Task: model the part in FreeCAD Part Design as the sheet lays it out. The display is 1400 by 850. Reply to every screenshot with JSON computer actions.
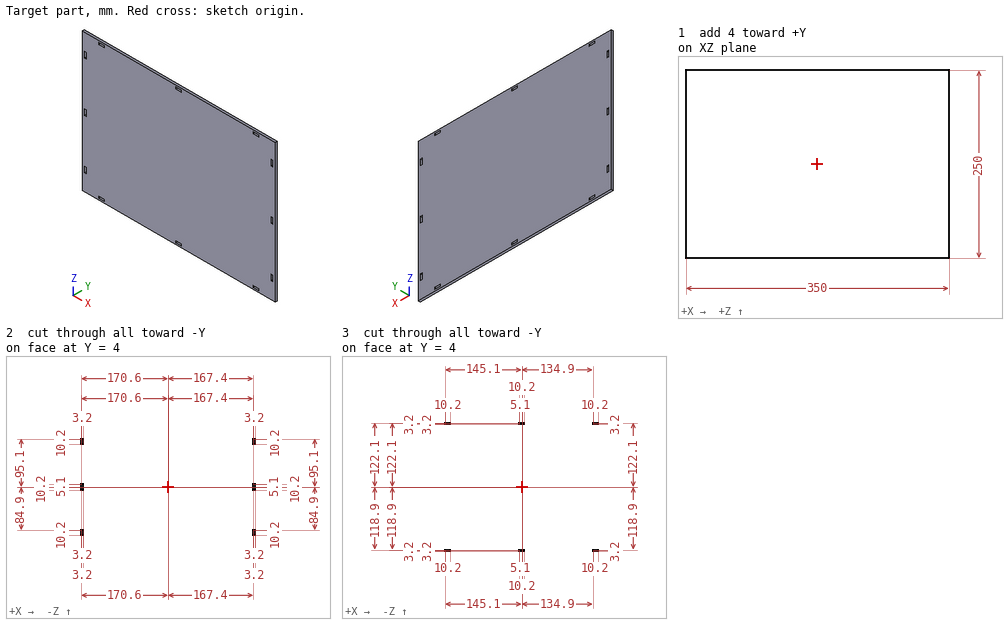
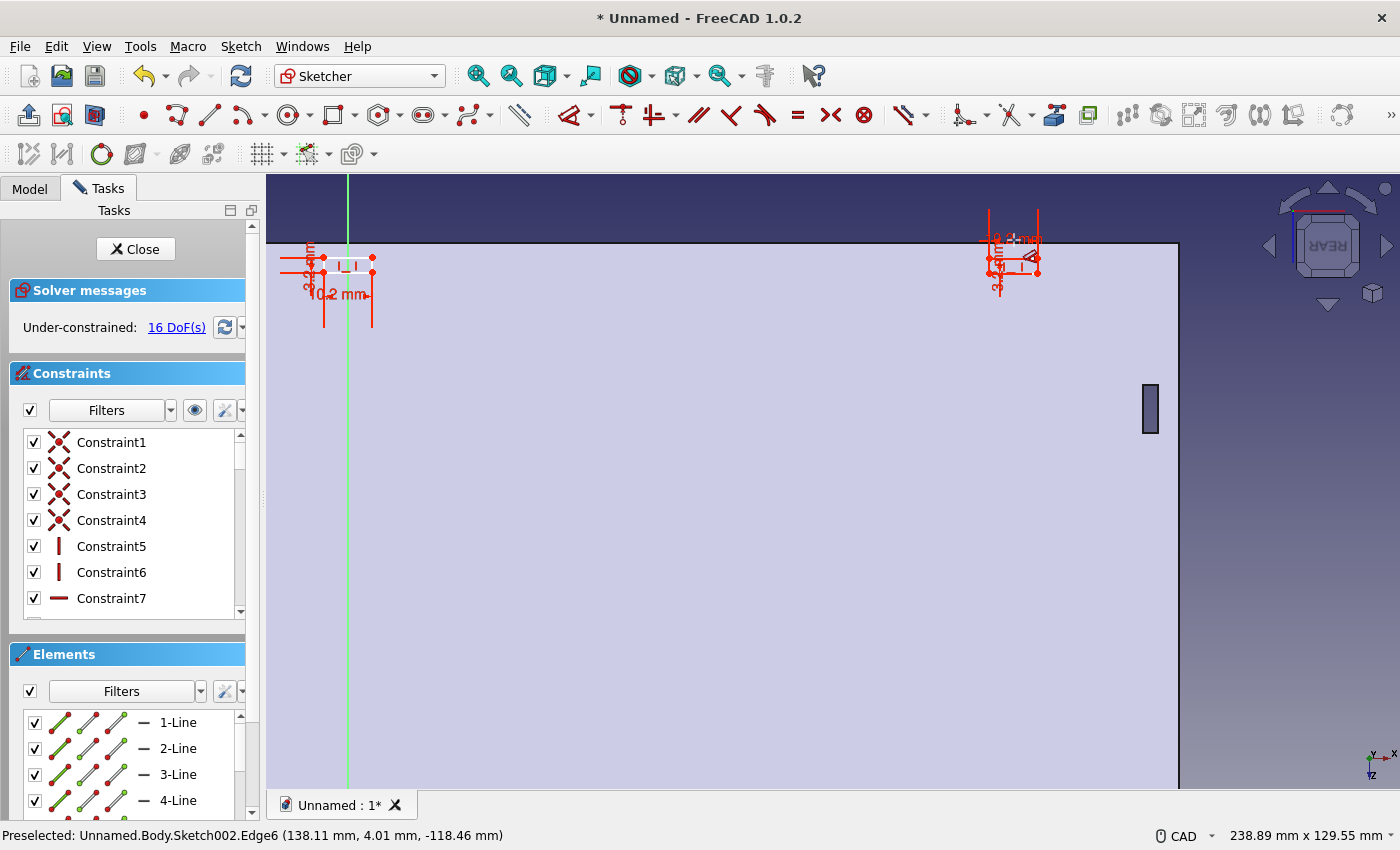
{"action": "scroll", "coordinate": [1007, 275], "scroll_direction": "down", "scroll_amount": 5}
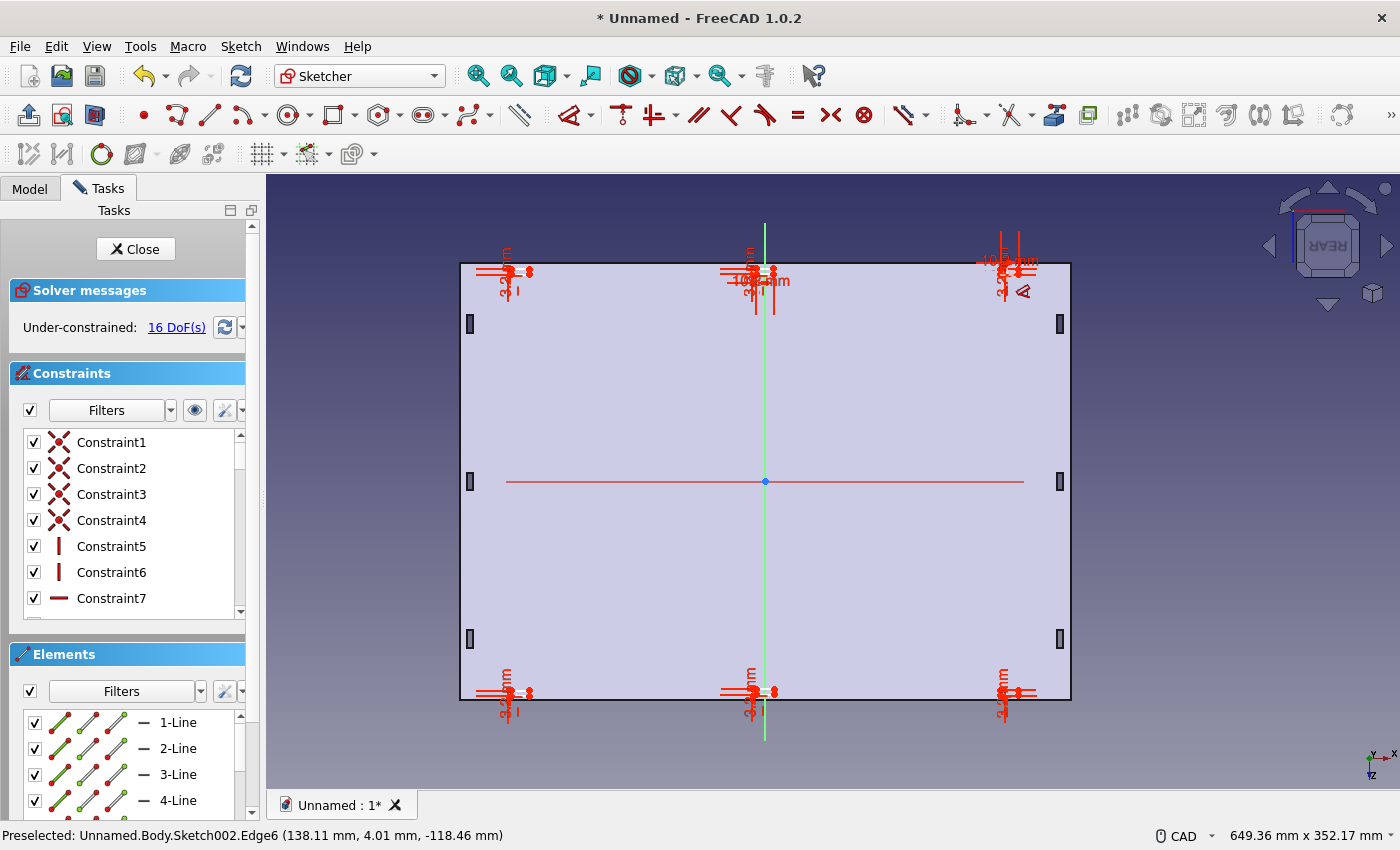
{"action": "scroll", "coordinate": [517, 275], "scroll_direction": "up", "scroll_amount": 5}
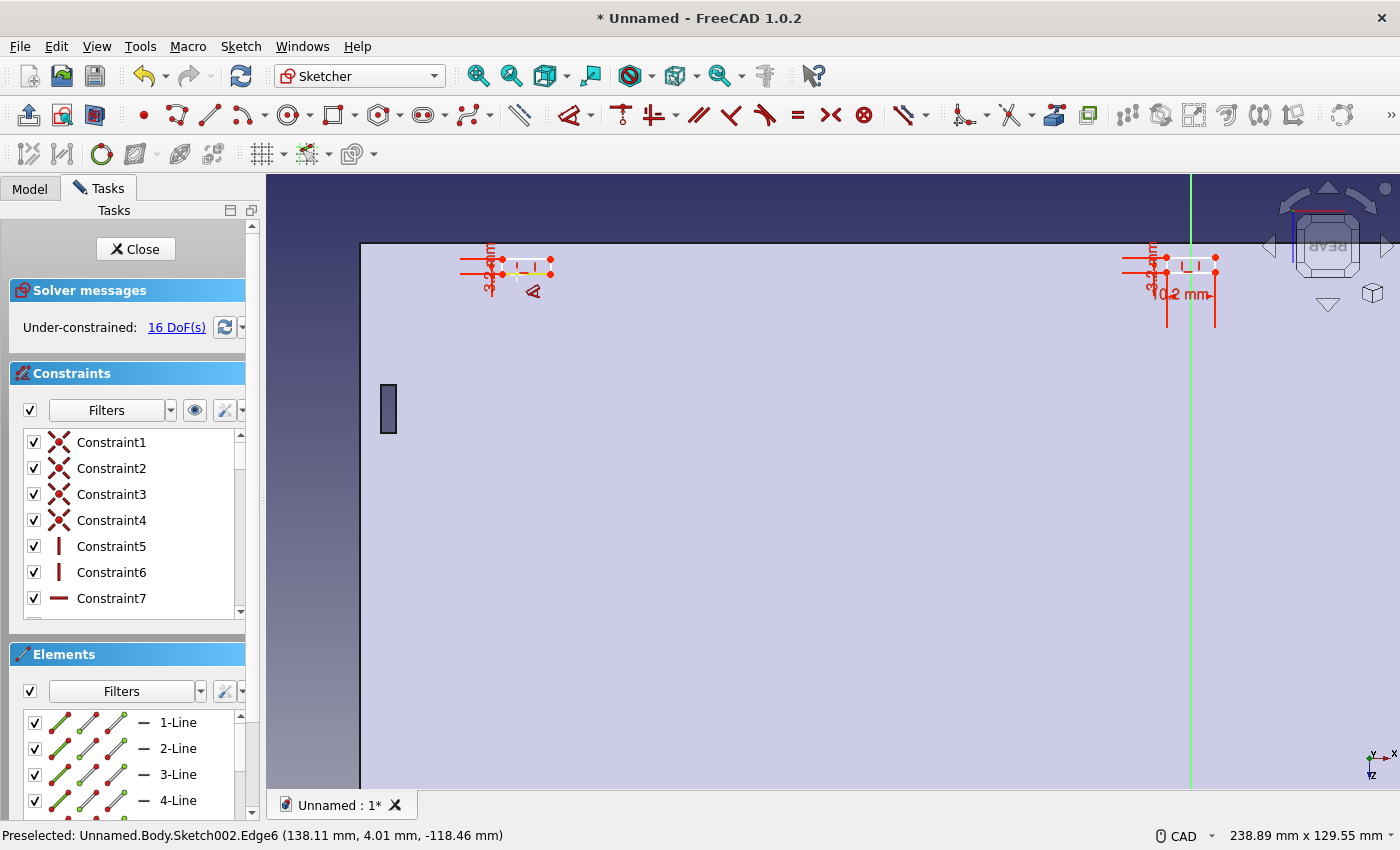
{"action": "left_click", "coordinate": [517, 274]}
{"action": "left_click", "coordinate": [526, 240]}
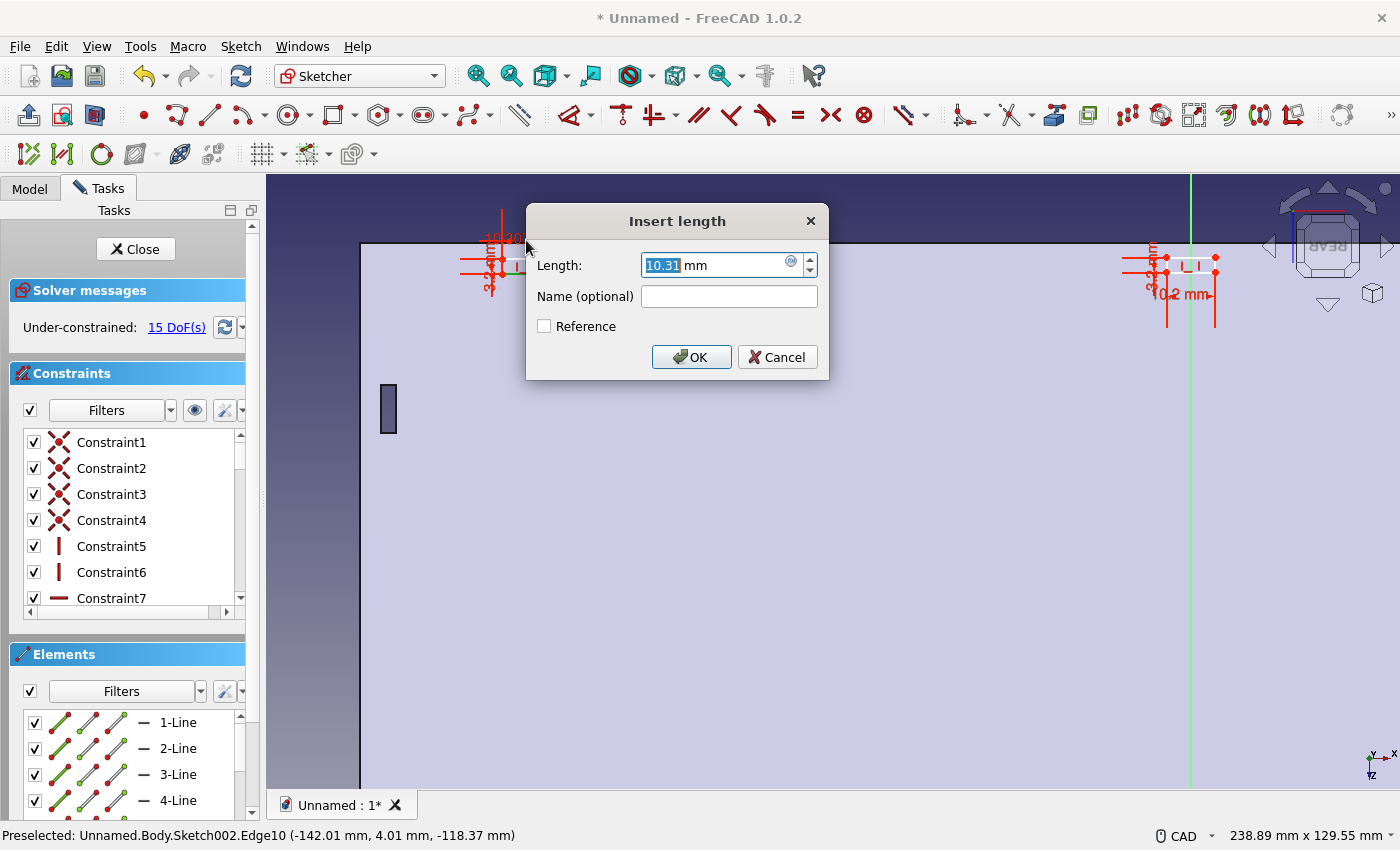
{"action": "type", "text": "10.2"}
{"action": "key", "text": "Return"}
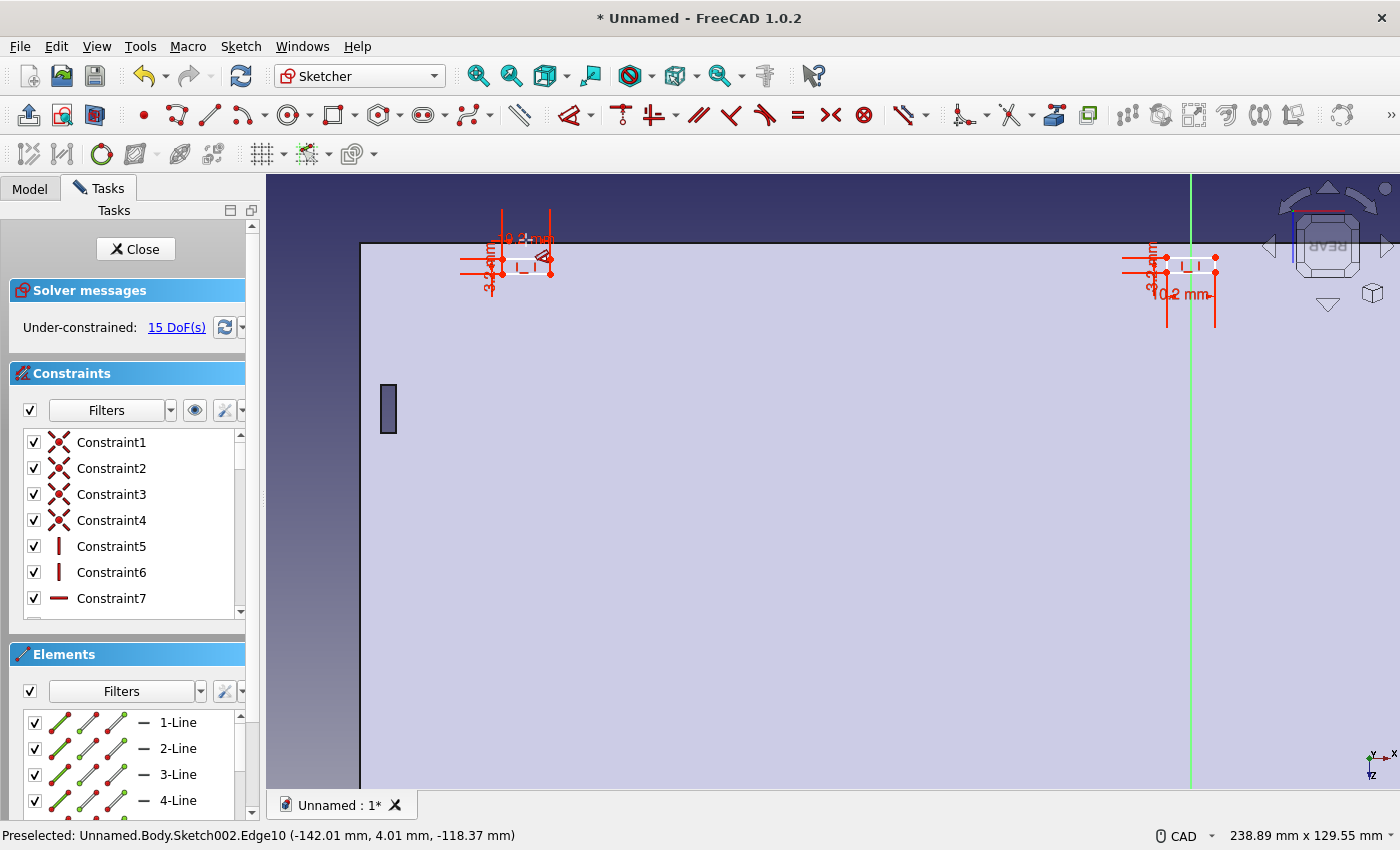
{"action": "scroll", "coordinate": [516, 275], "scroll_direction": "down", "scroll_amount": 5}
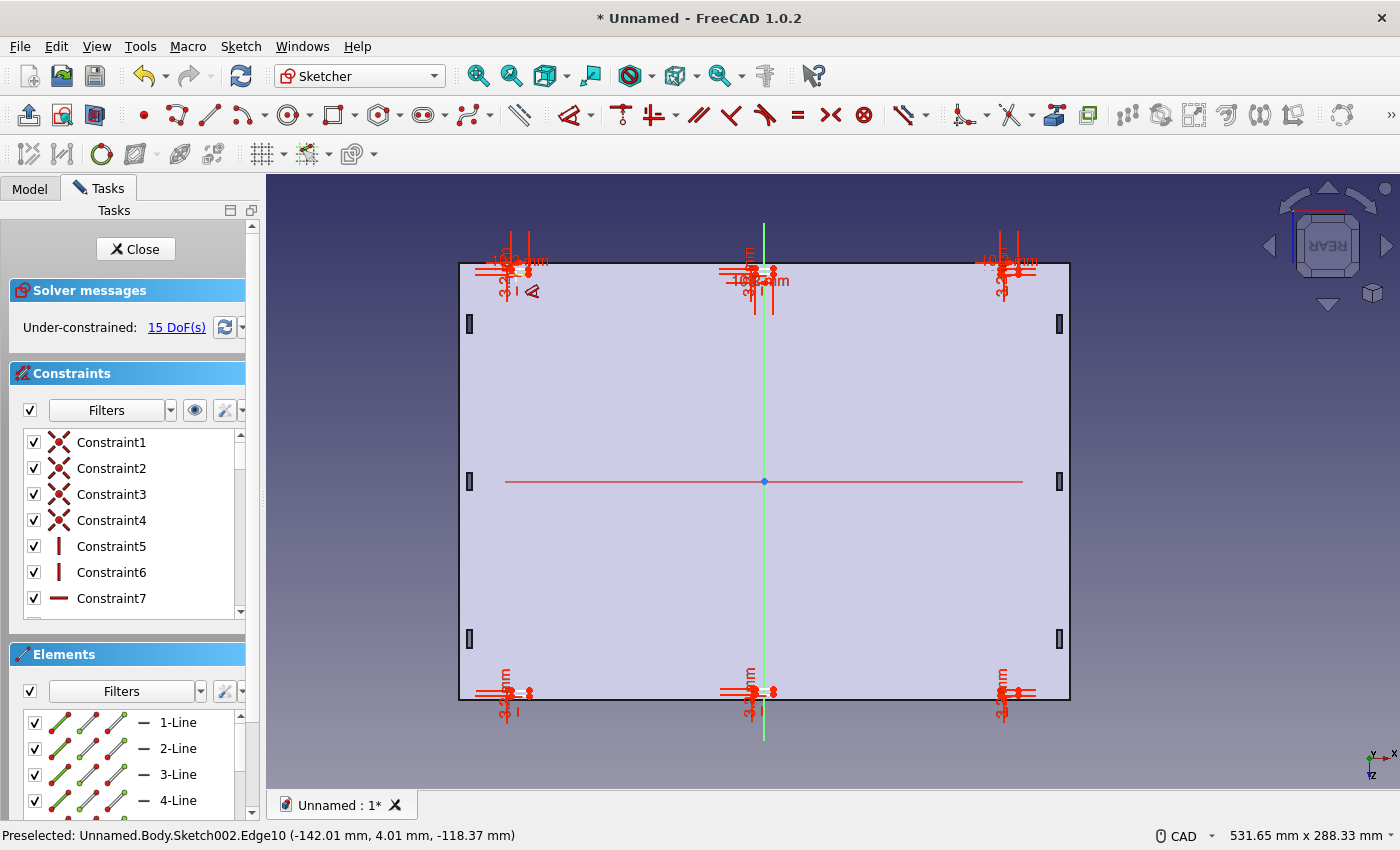
{"action": "scroll", "coordinate": [516, 696], "scroll_direction": "up", "scroll_amount": 5}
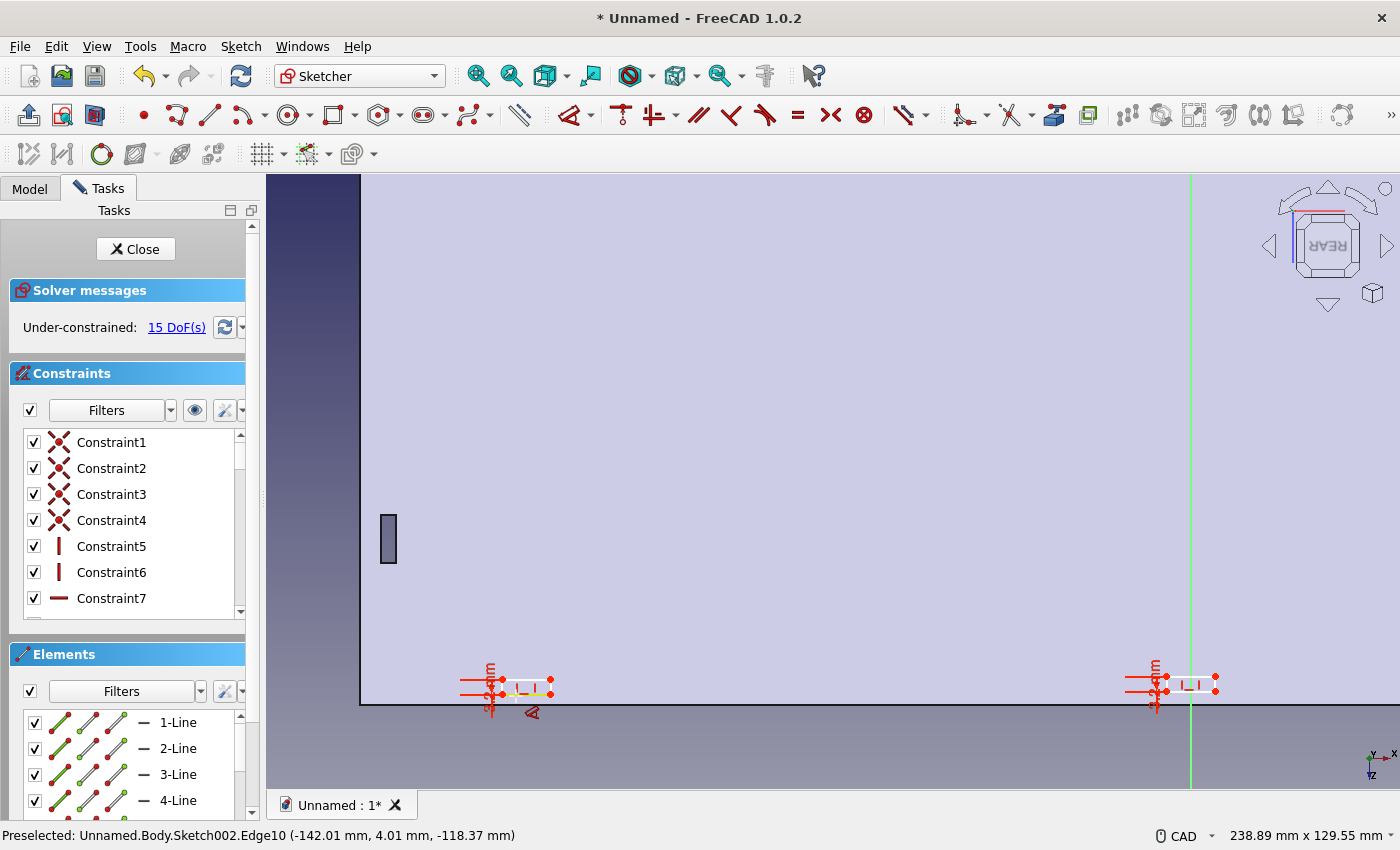
{"action": "left_click", "coordinate": [517, 695]}
{"action": "left_click", "coordinate": [526, 729]}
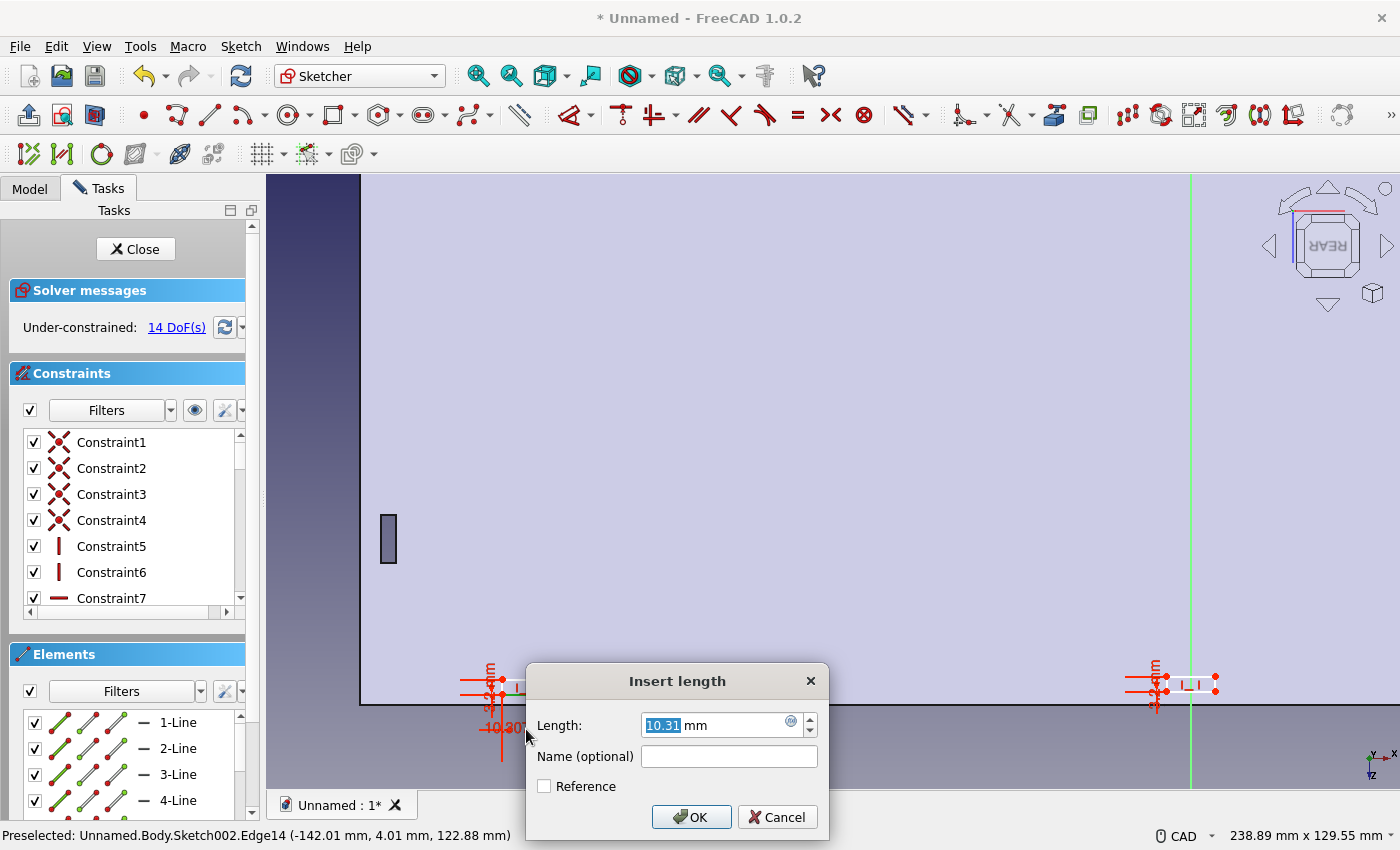
{"action": "type", "text": "10.2"}
{"action": "key", "text": "Return"}